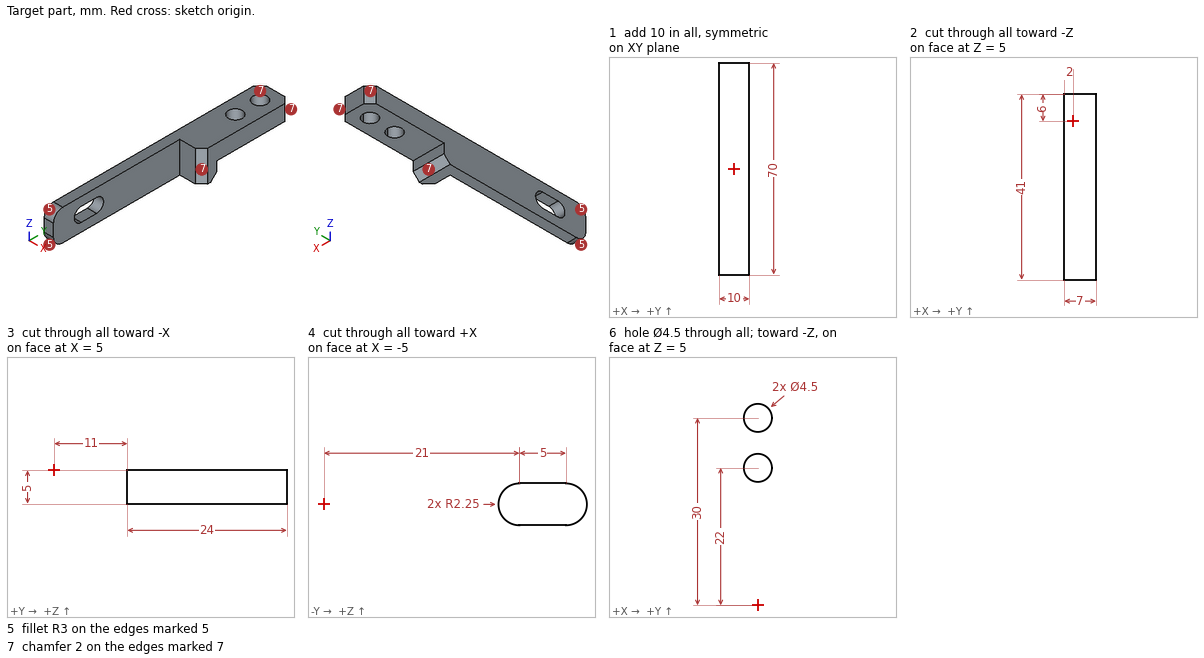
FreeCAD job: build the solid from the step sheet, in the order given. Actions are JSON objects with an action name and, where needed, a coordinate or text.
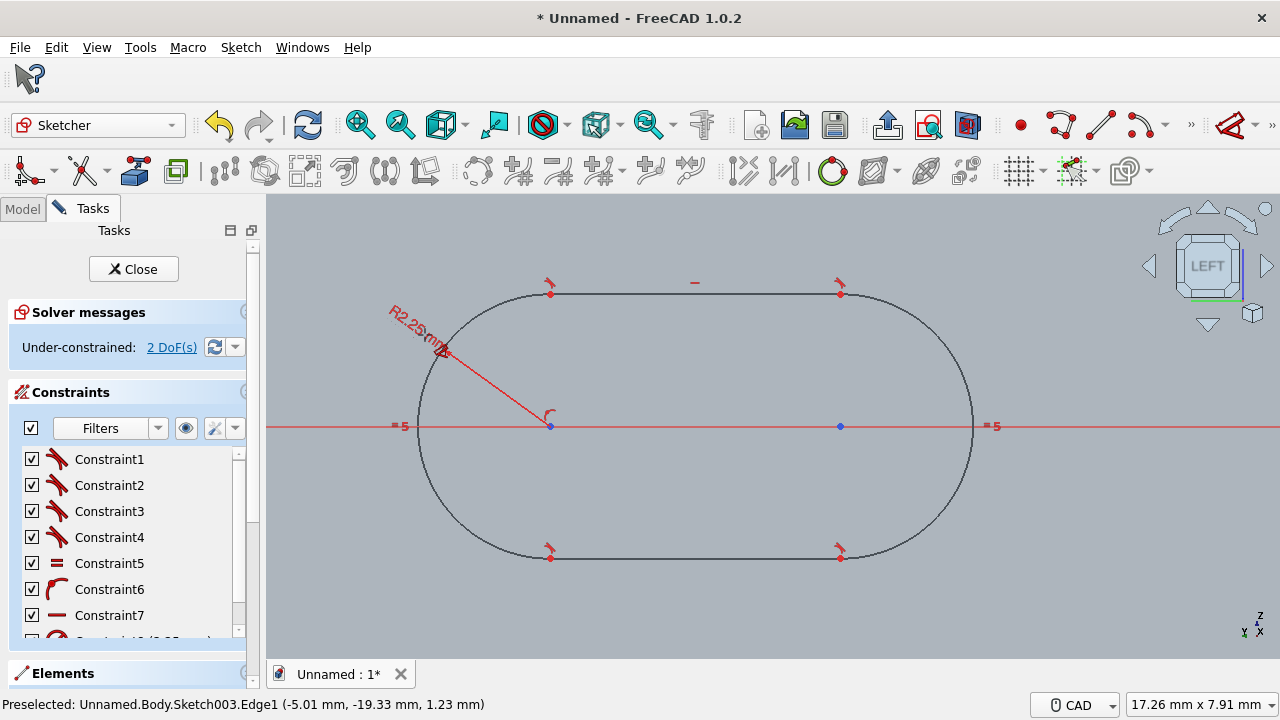
{"action": "left_click", "coordinate": [637, 294]}
{"action": "left_click", "coordinate": [696, 260]}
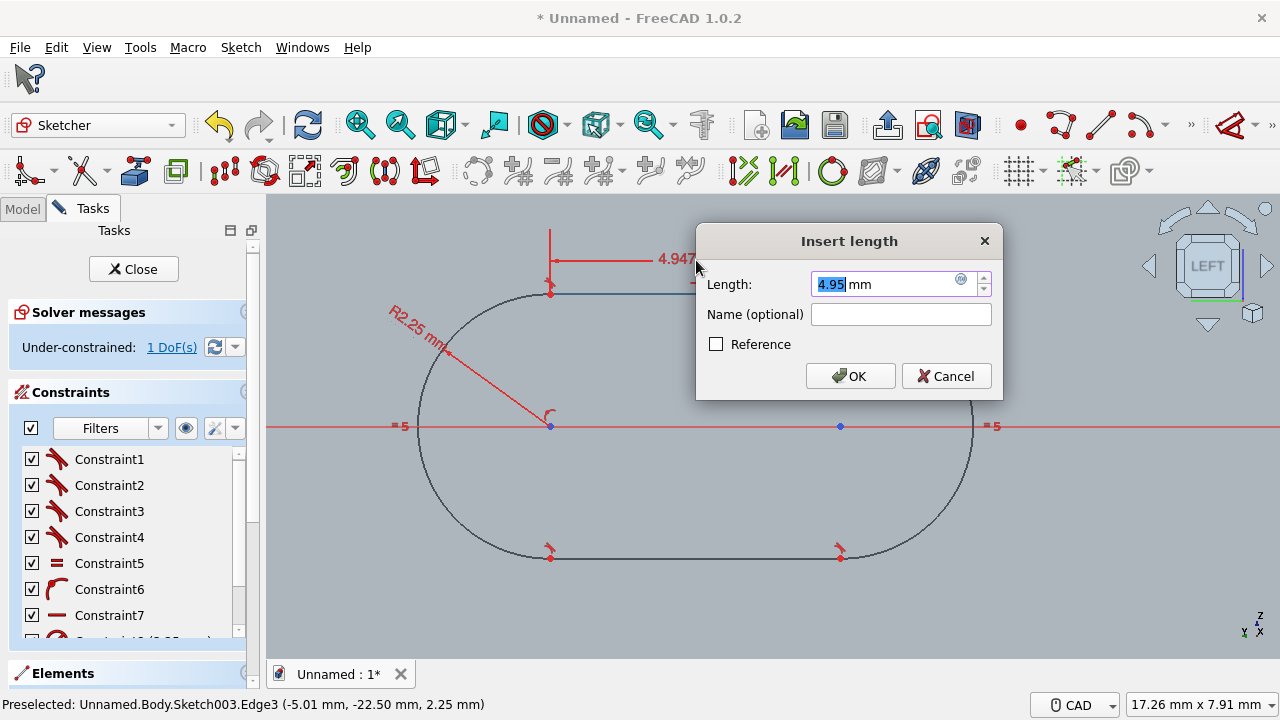
{"action": "type", "text": "5"}
{"action": "key", "text": "Return"}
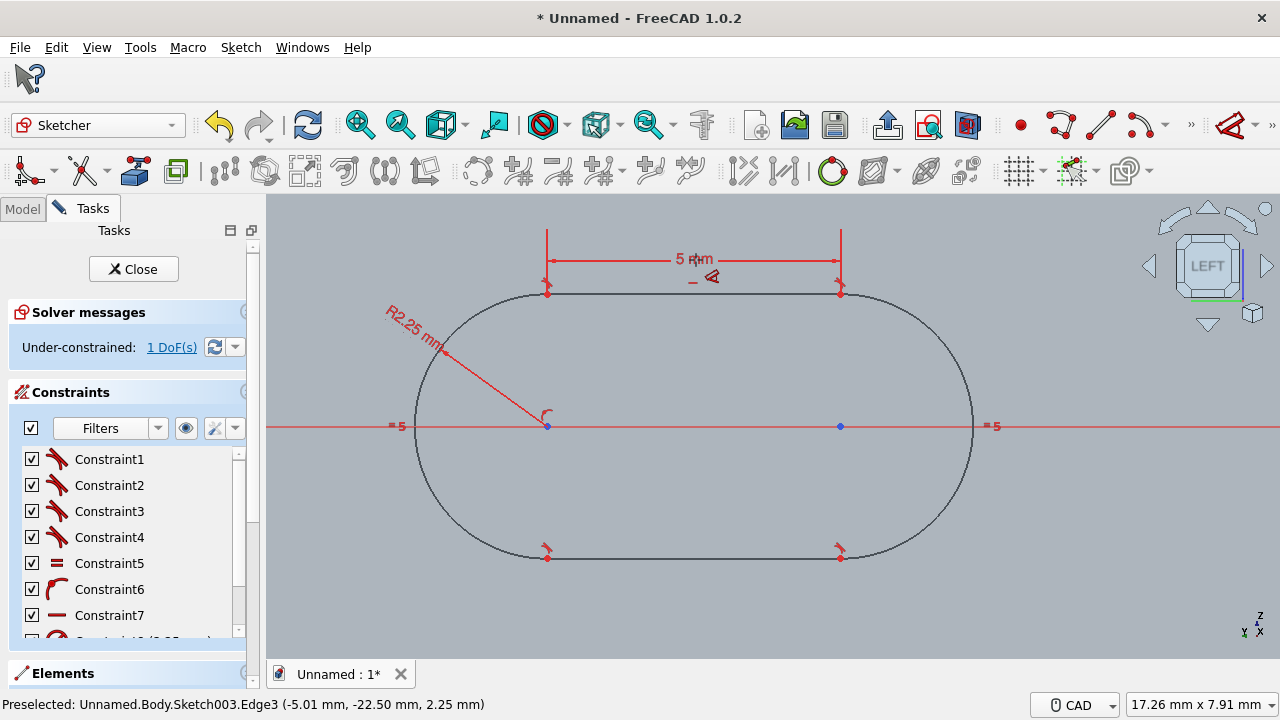
{"action": "left_click", "coordinate": [547, 294]}
{"action": "left_click", "coordinate": [421, 260]}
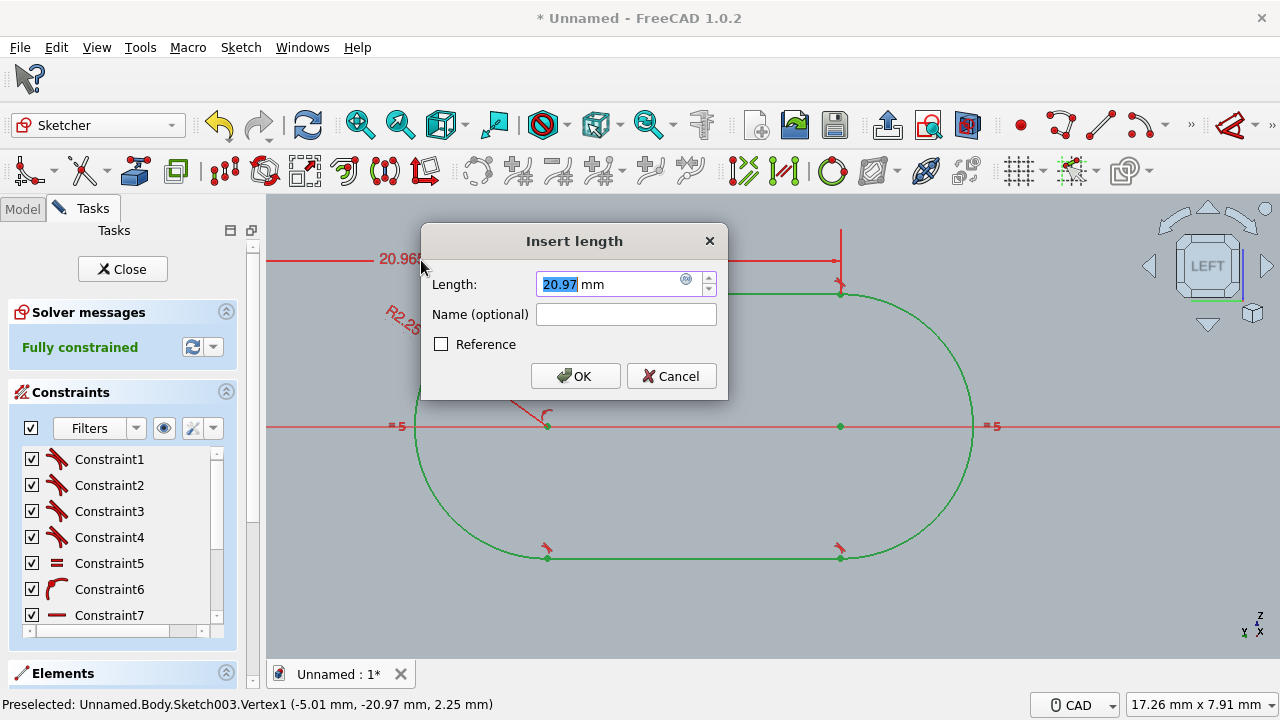
{"action": "type", "text": "21"}
{"action": "key", "text": "Return"}
{"action": "key", "text": "Escape"}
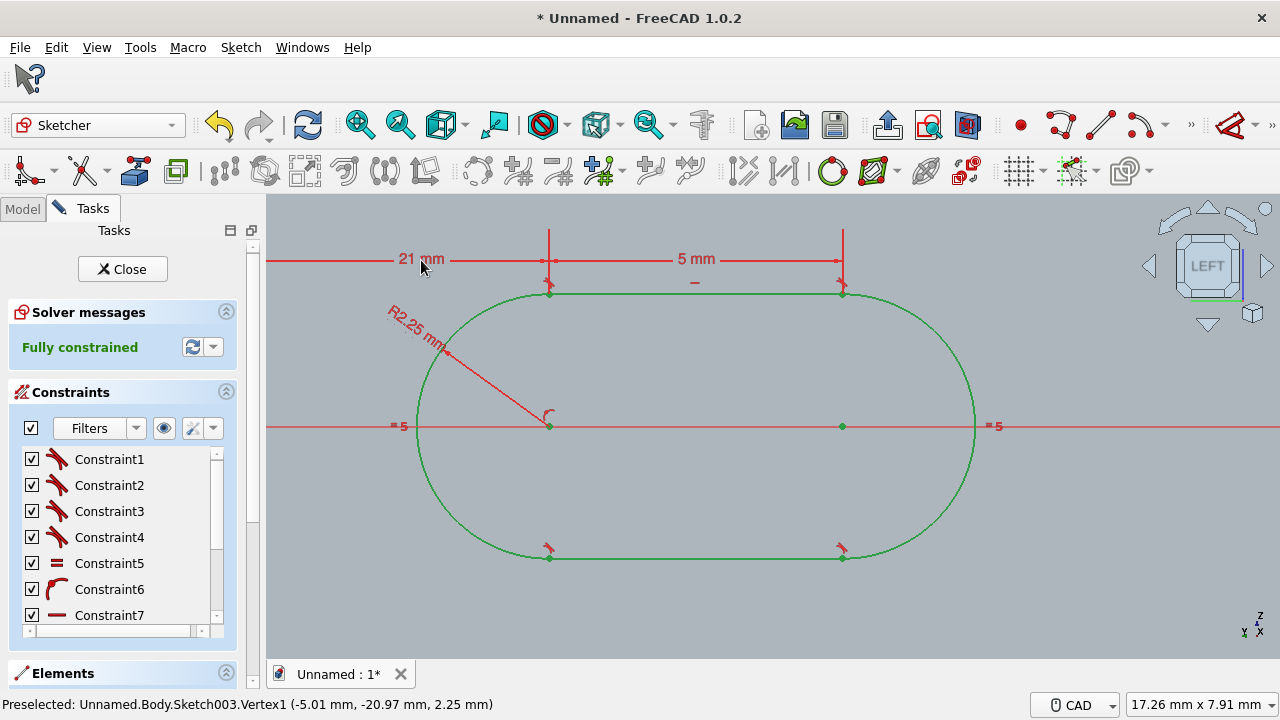
{"action": "left_click", "coordinate": [123, 269]}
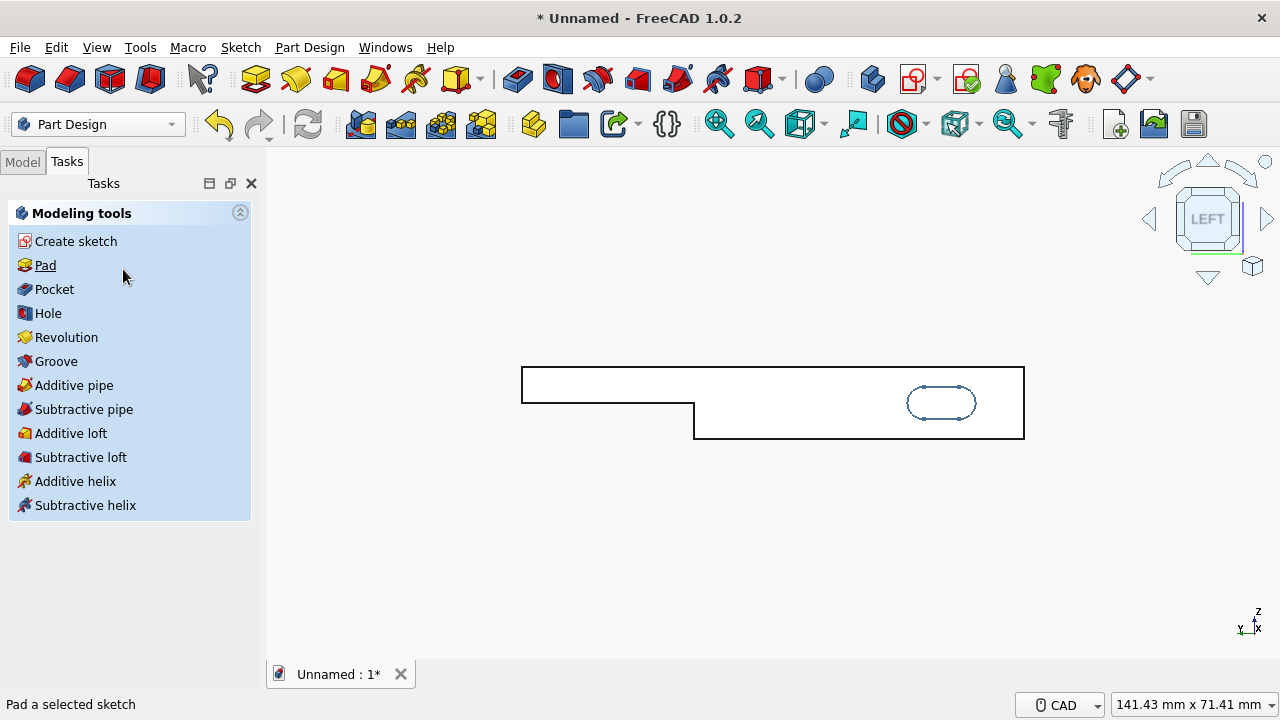
{"action": "left_click", "coordinate": [518, 80]}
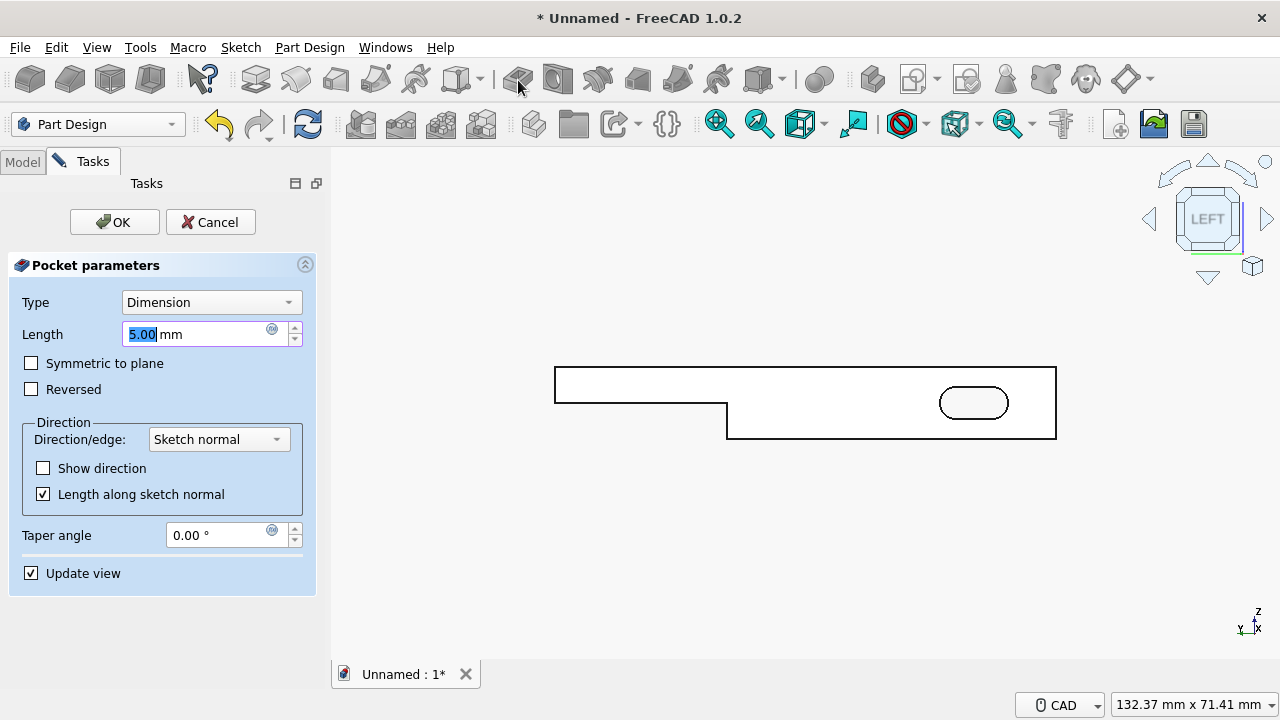
{"action": "left_click", "coordinate": [212, 302]}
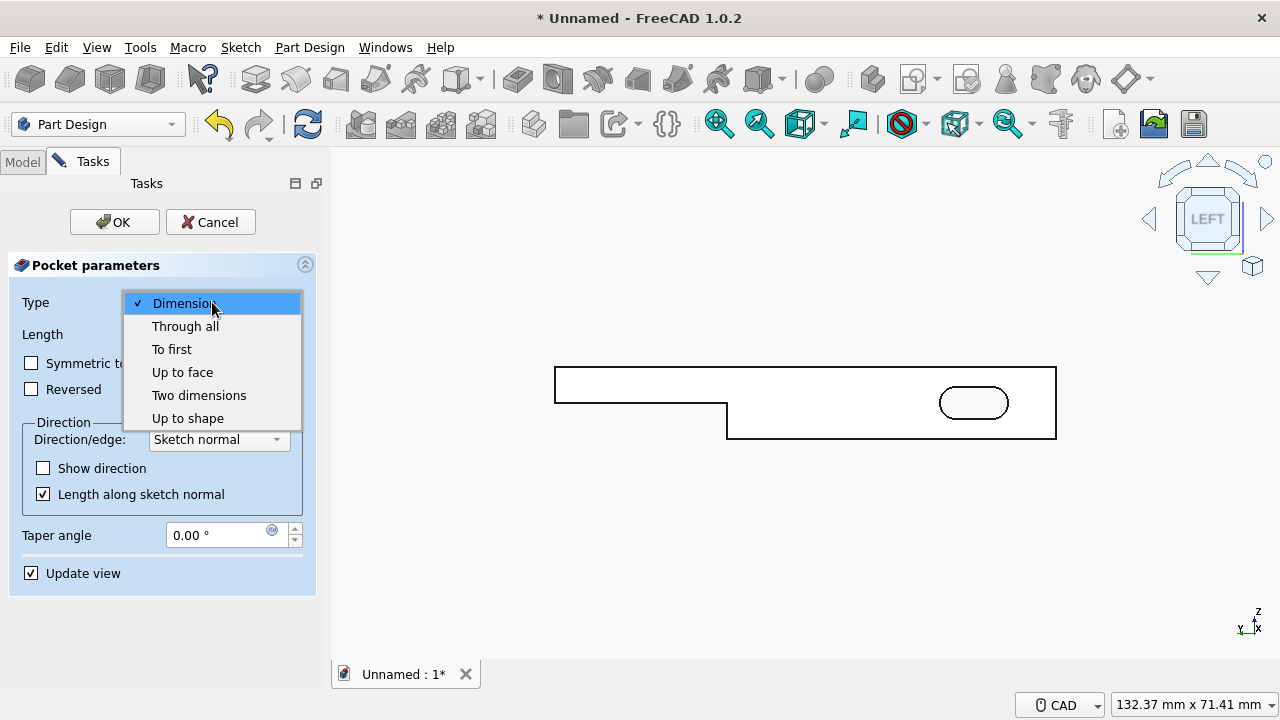
{"action": "left_click", "coordinate": [212, 326]}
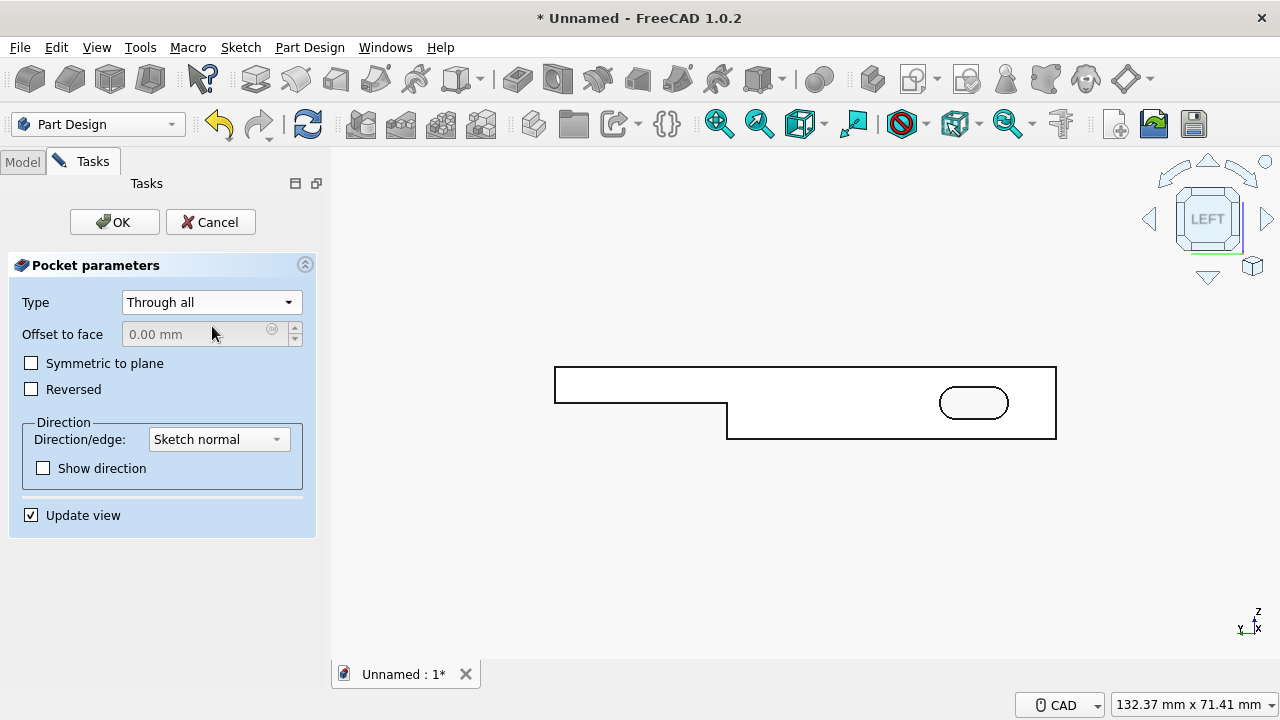
{"action": "left_click", "coordinate": [115, 222]}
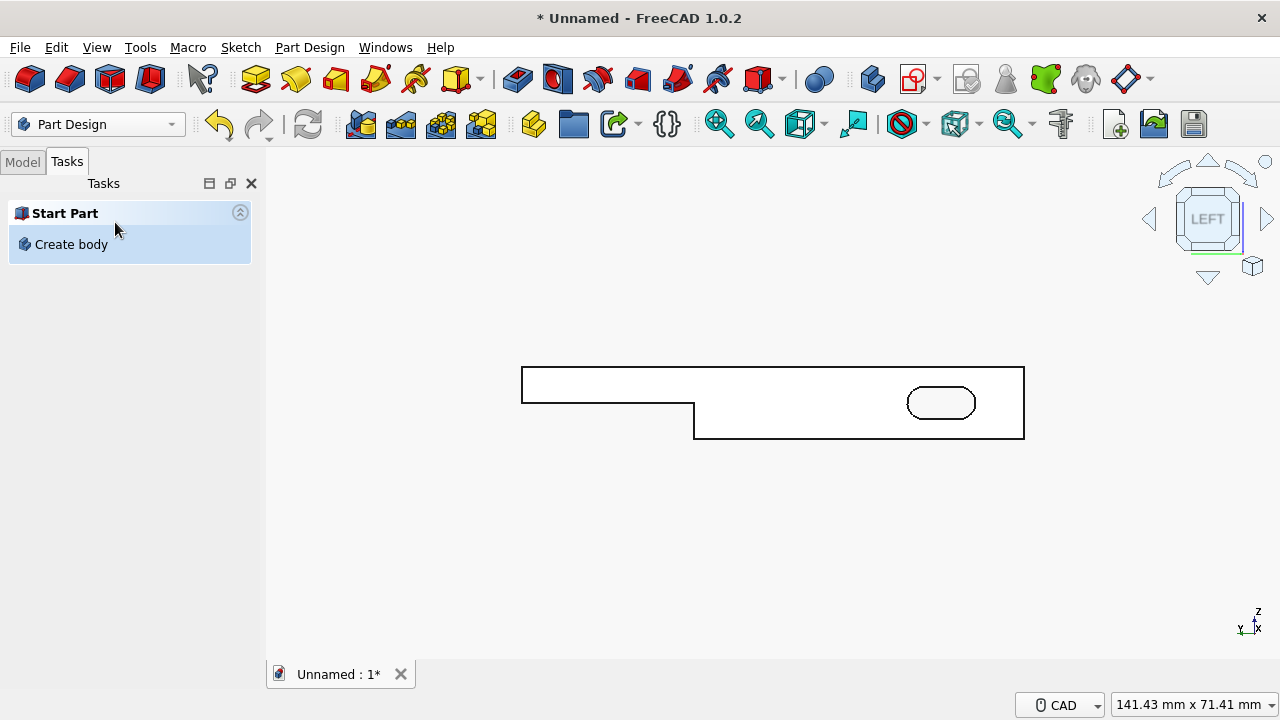
{"action": "scroll", "coordinate": [1024, 366], "scroll_direction": "up", "scroll_amount": 4}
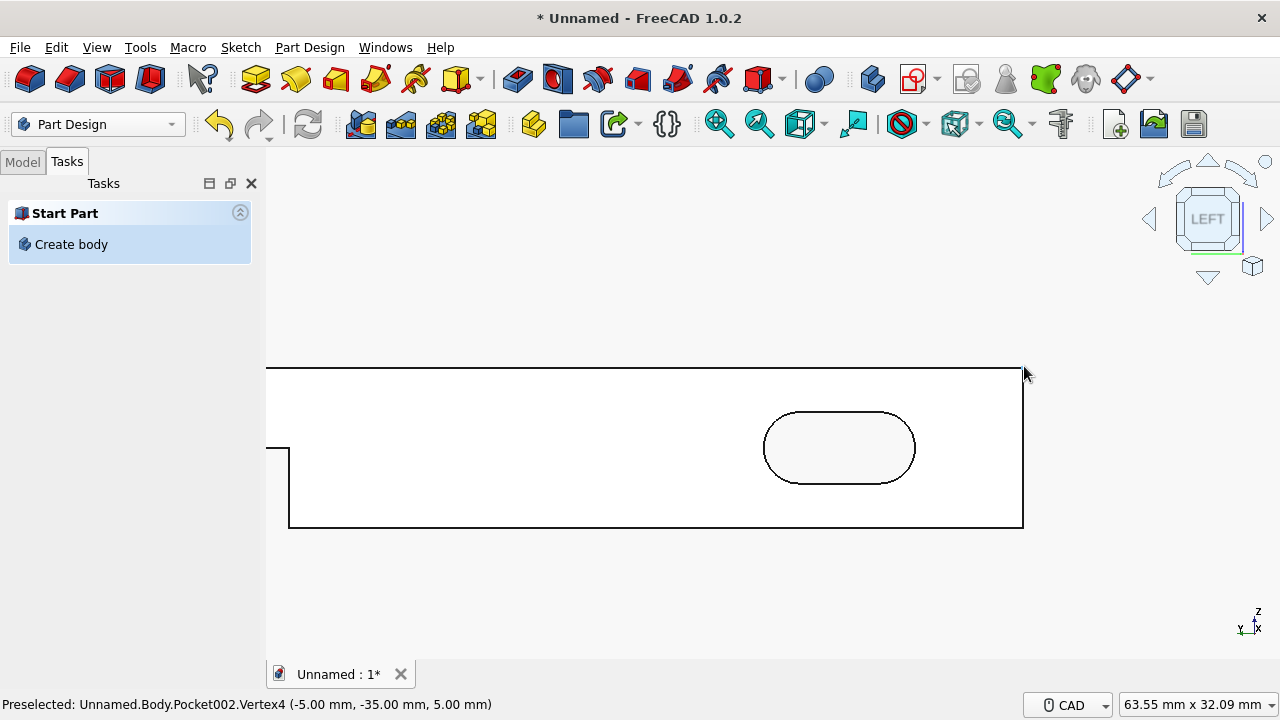
{"action": "key", "text": "v f"}